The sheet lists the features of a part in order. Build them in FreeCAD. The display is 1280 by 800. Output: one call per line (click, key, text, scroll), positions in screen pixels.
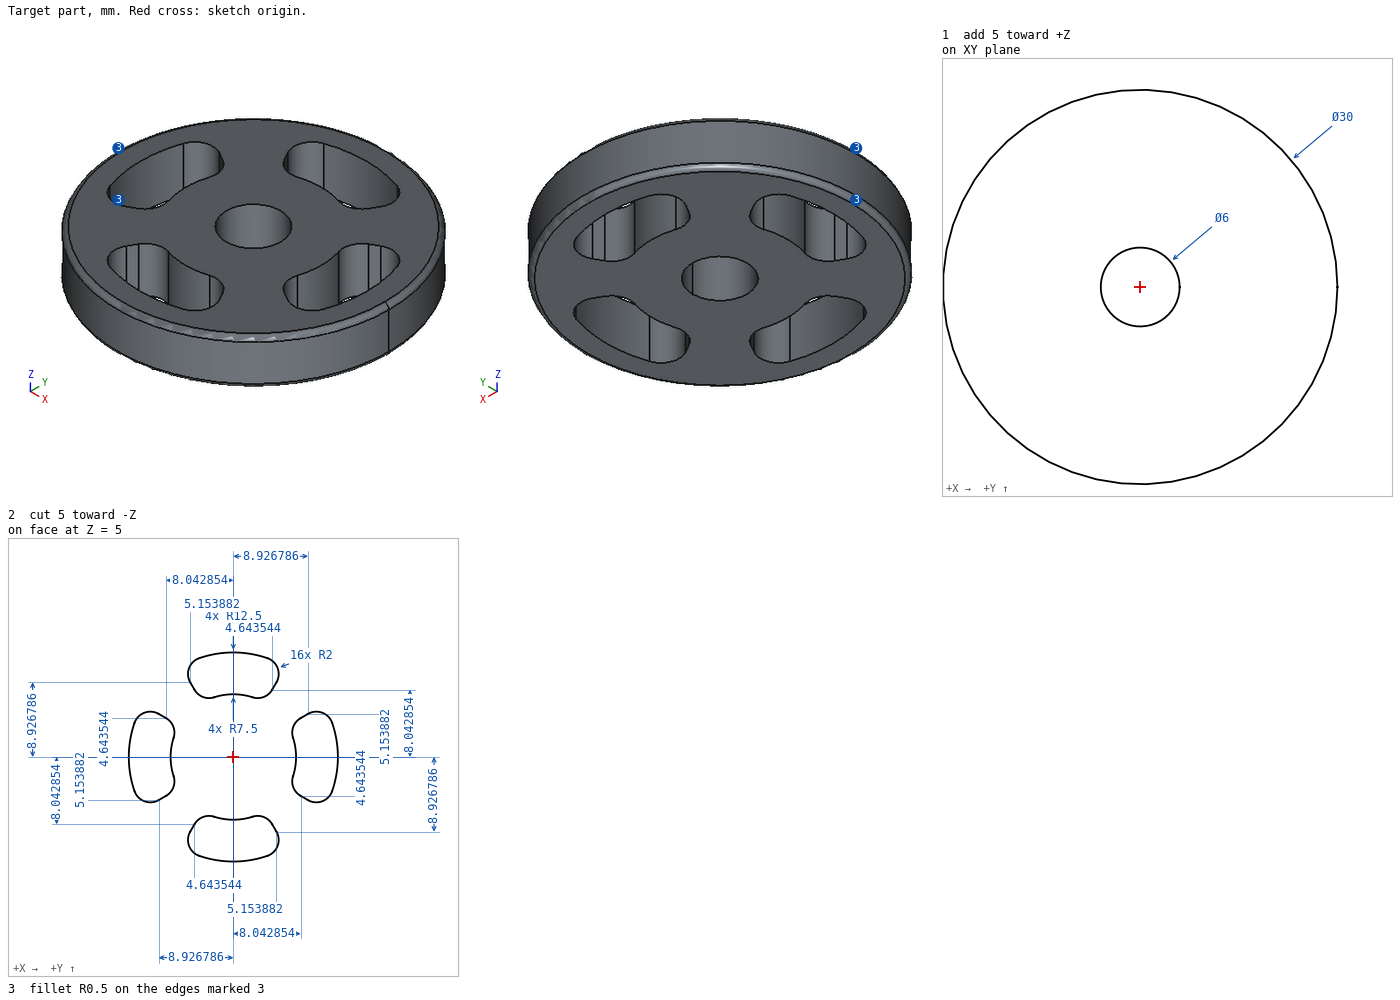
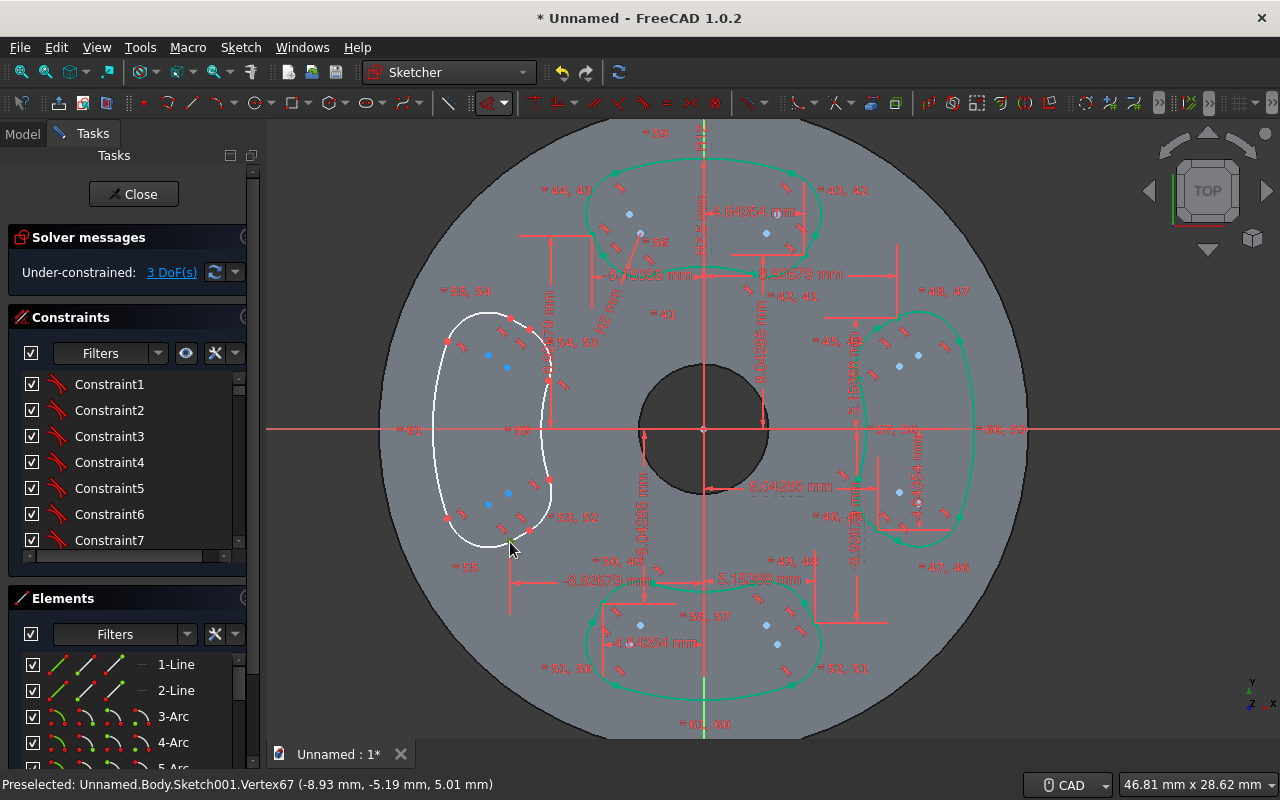
click(506, 104)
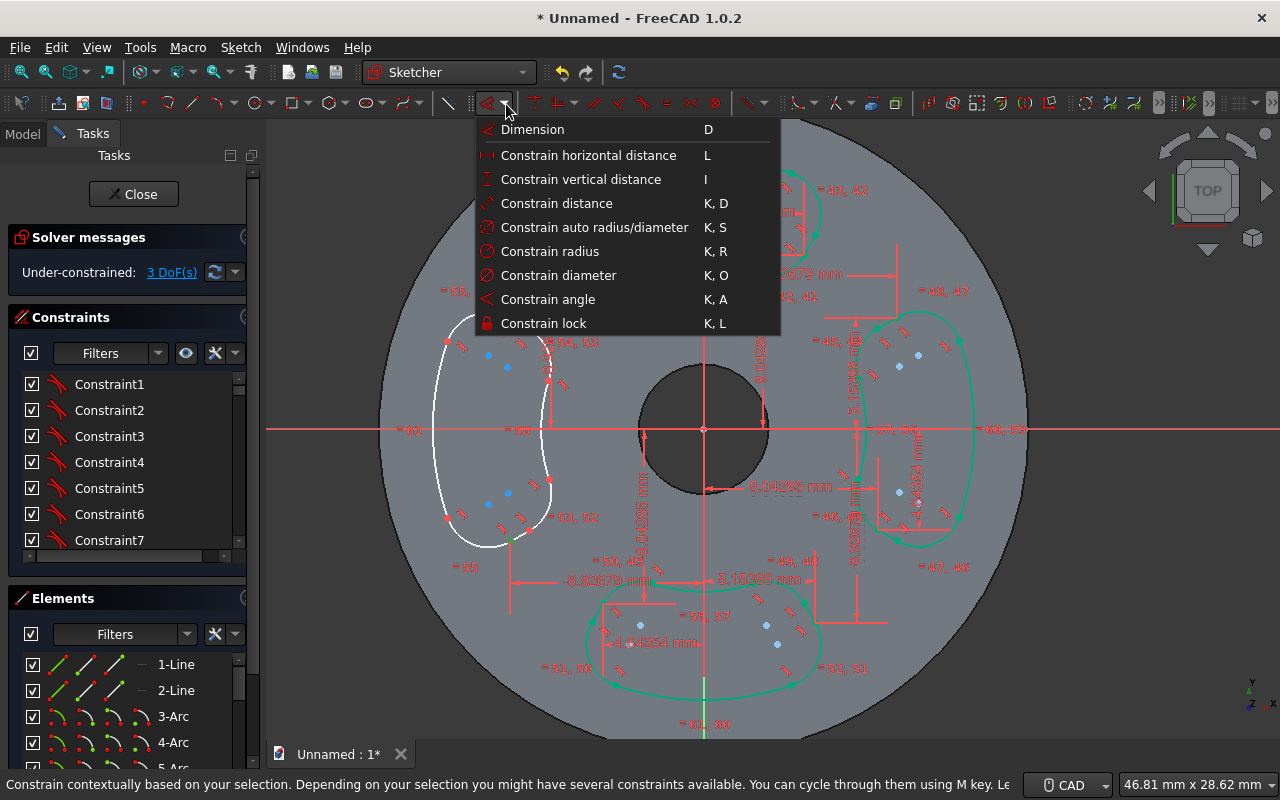
click(628, 179)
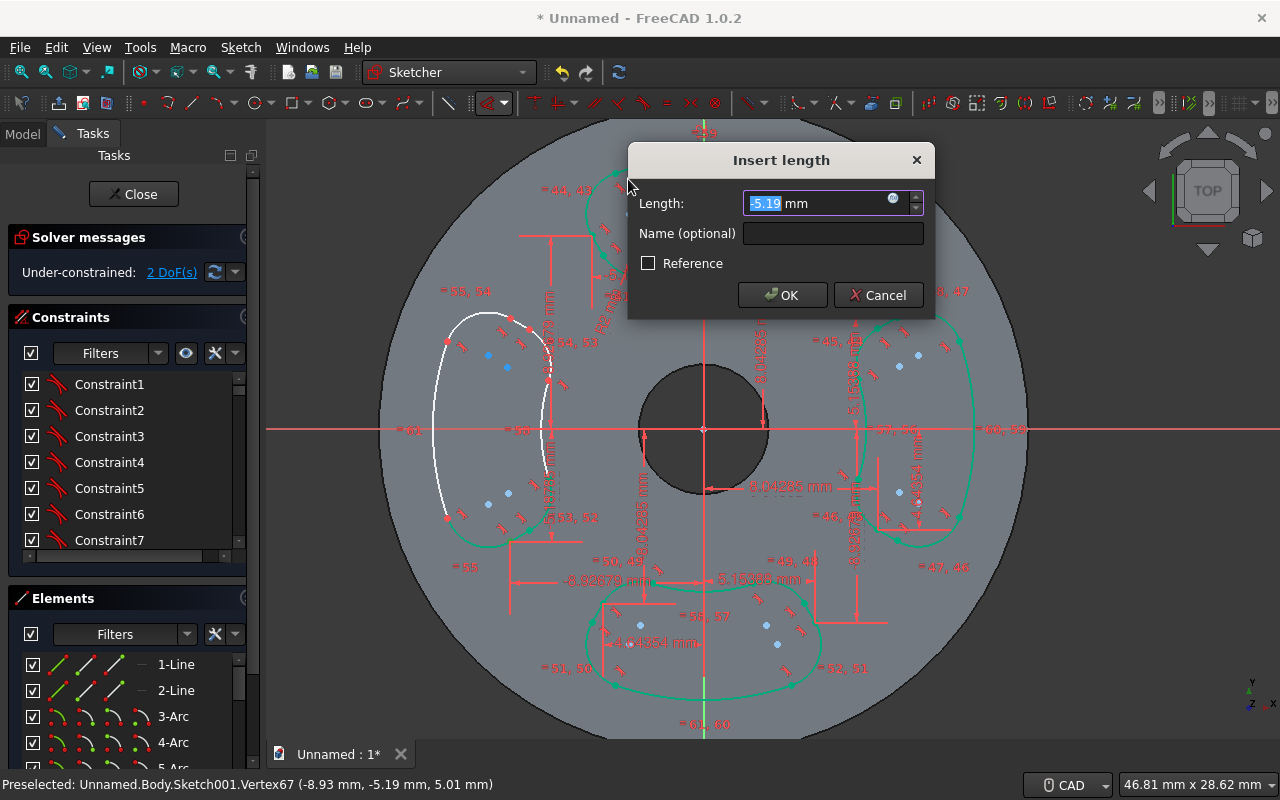
text(-5.153882)
key(Return)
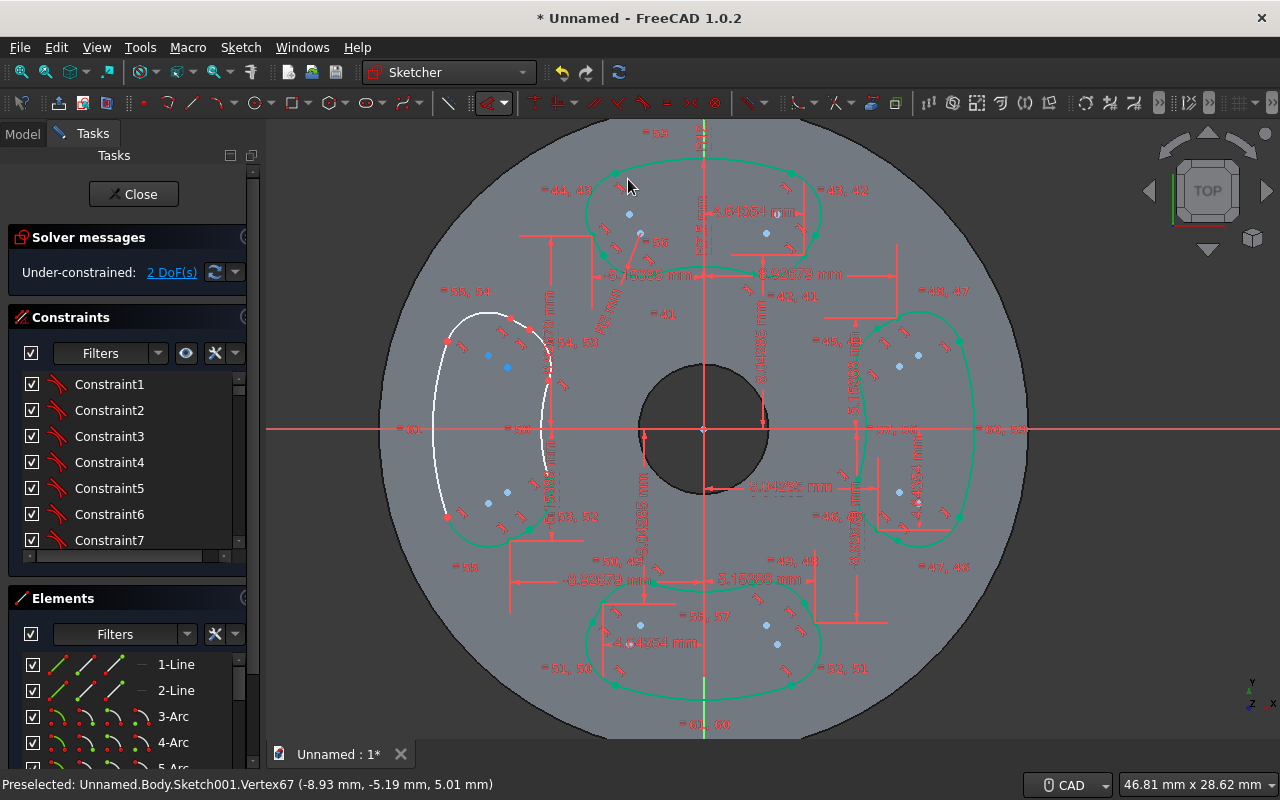
click(529, 330)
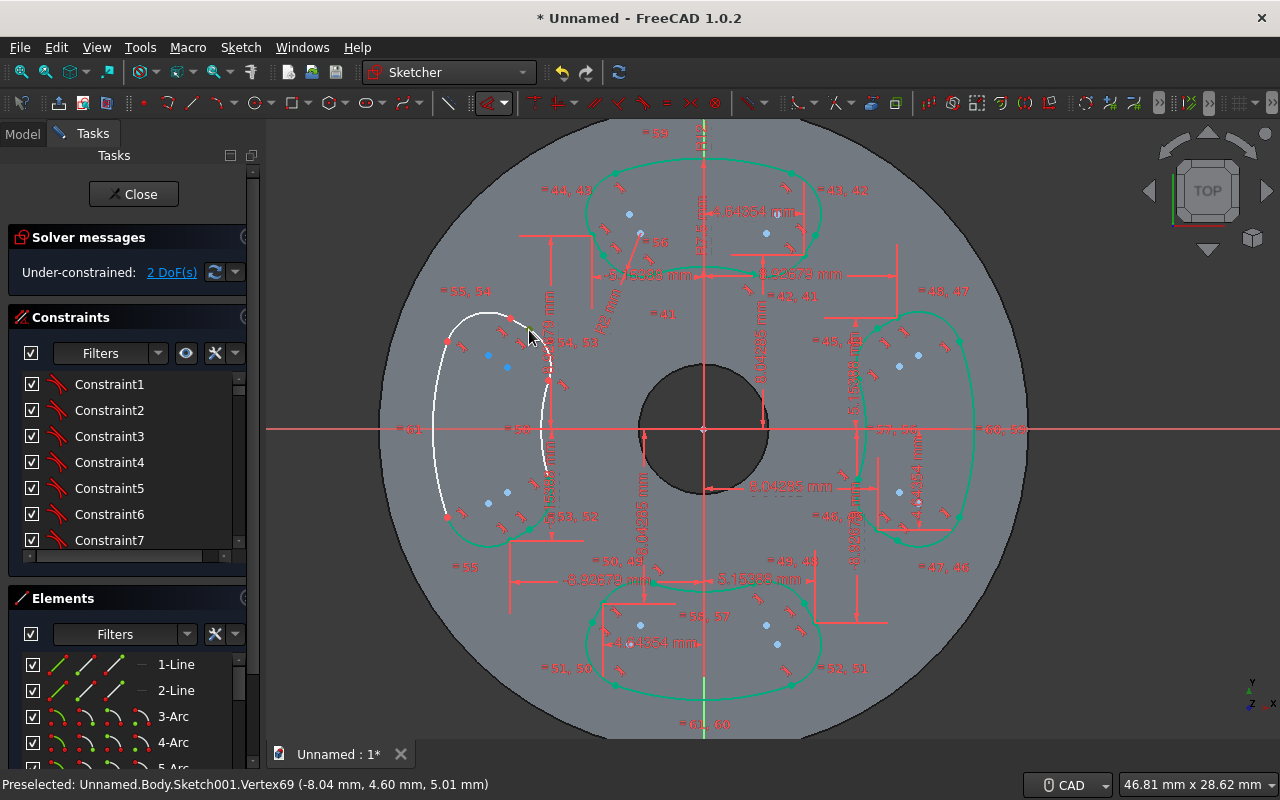
click(506, 104)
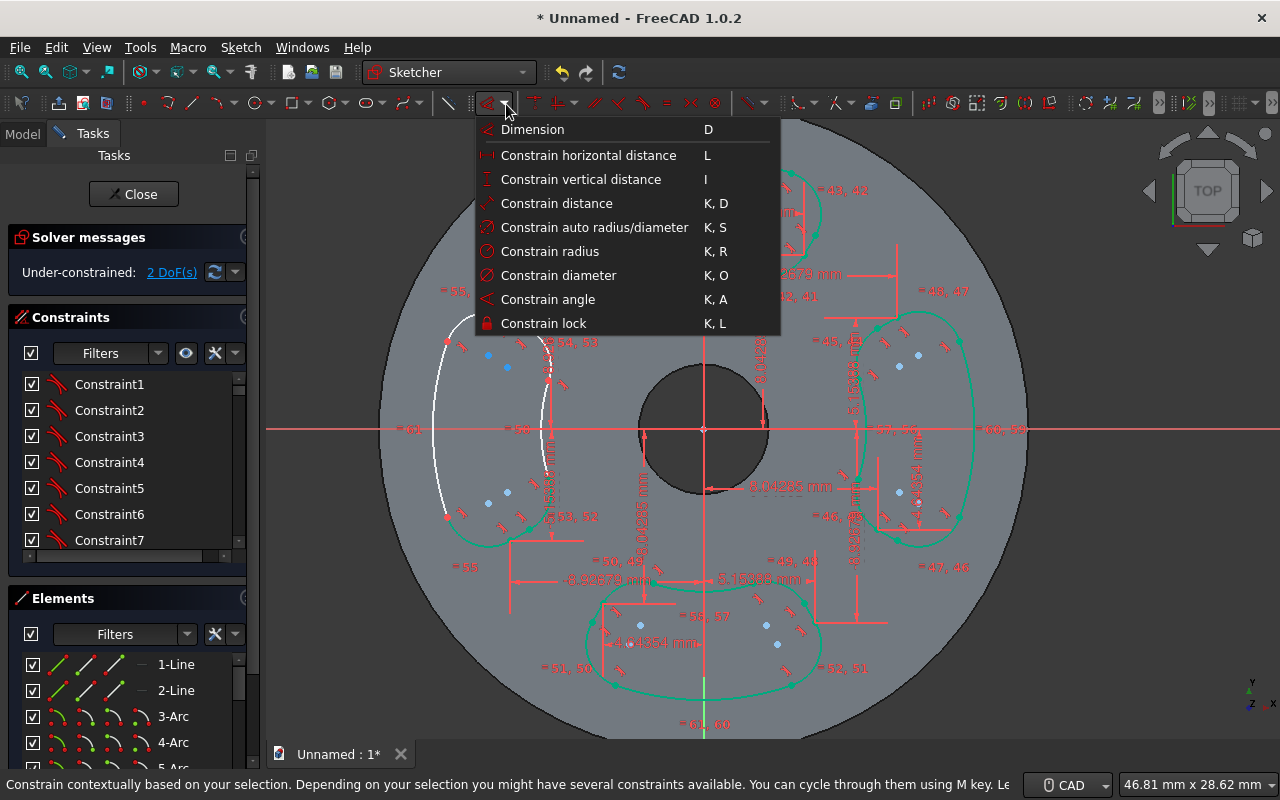
click(628, 155)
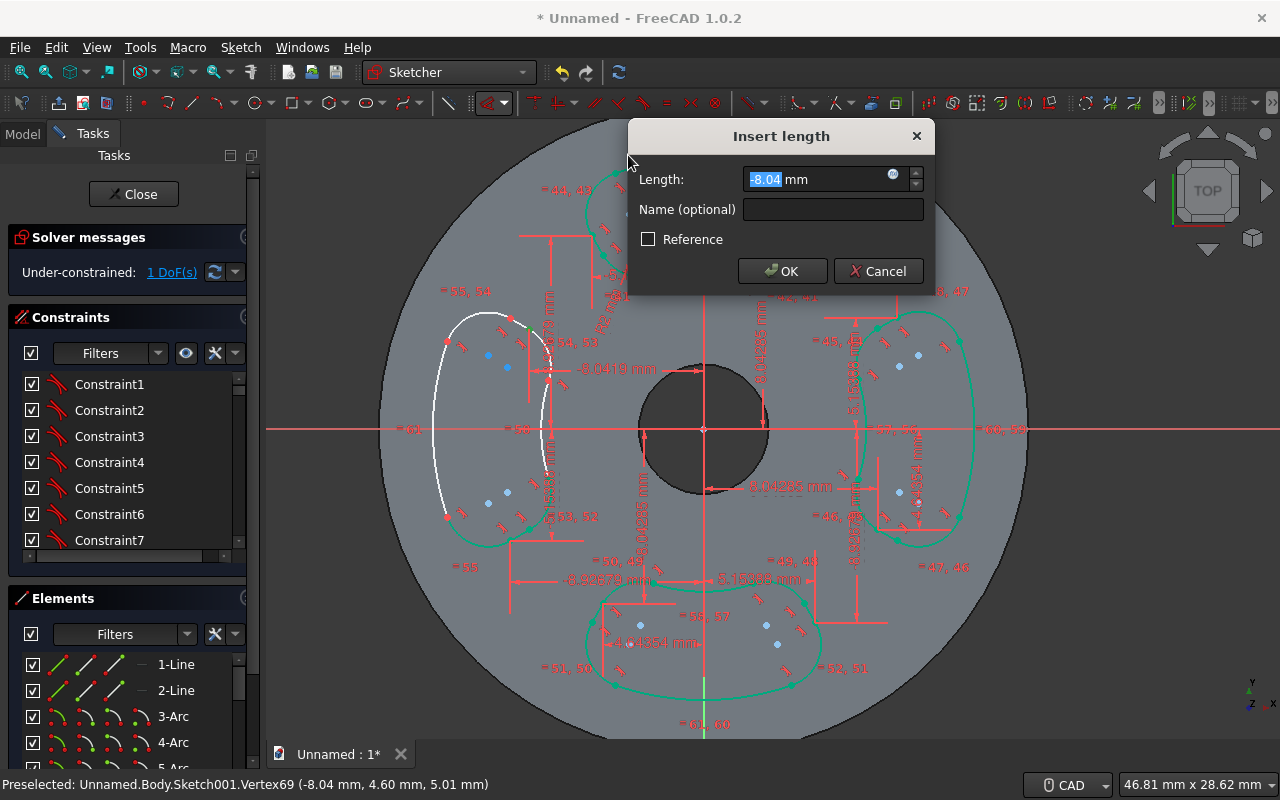
text(-8.042854)
key(Return)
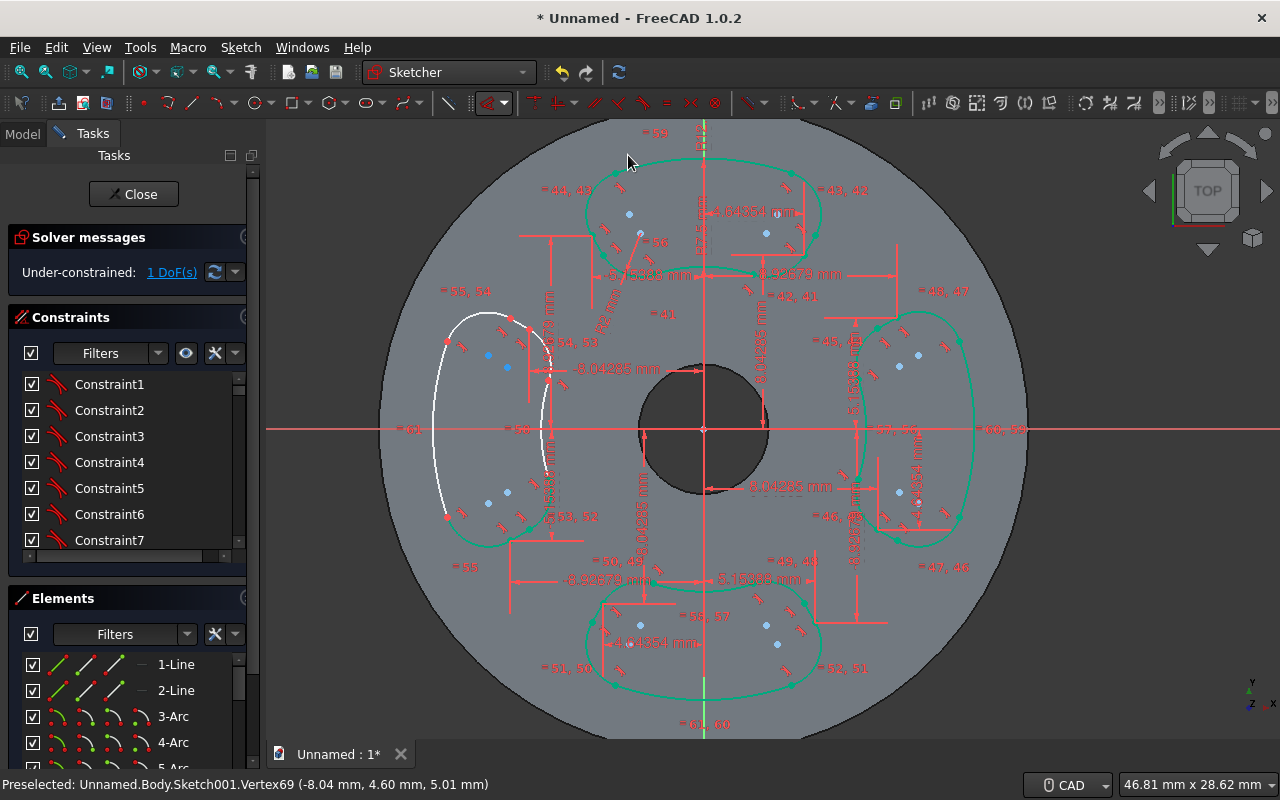
click(529, 330)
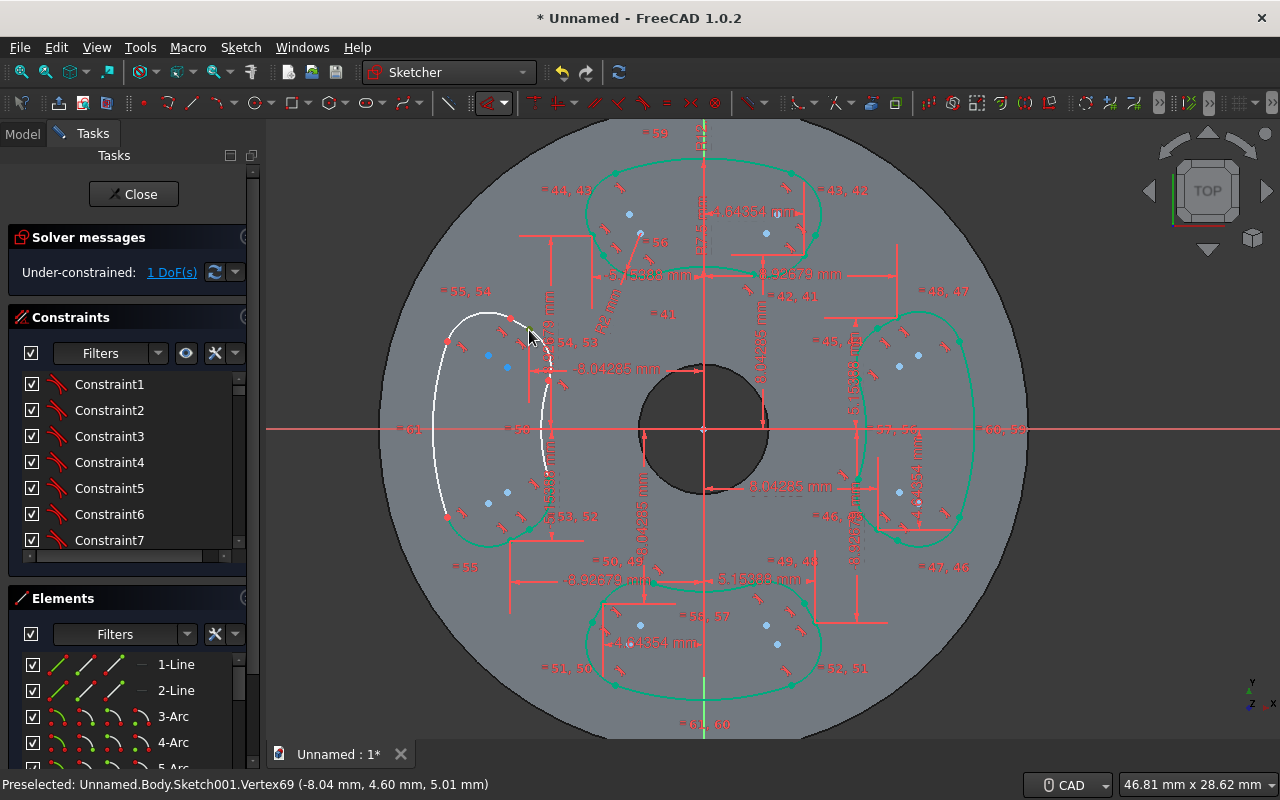
click(506, 104)